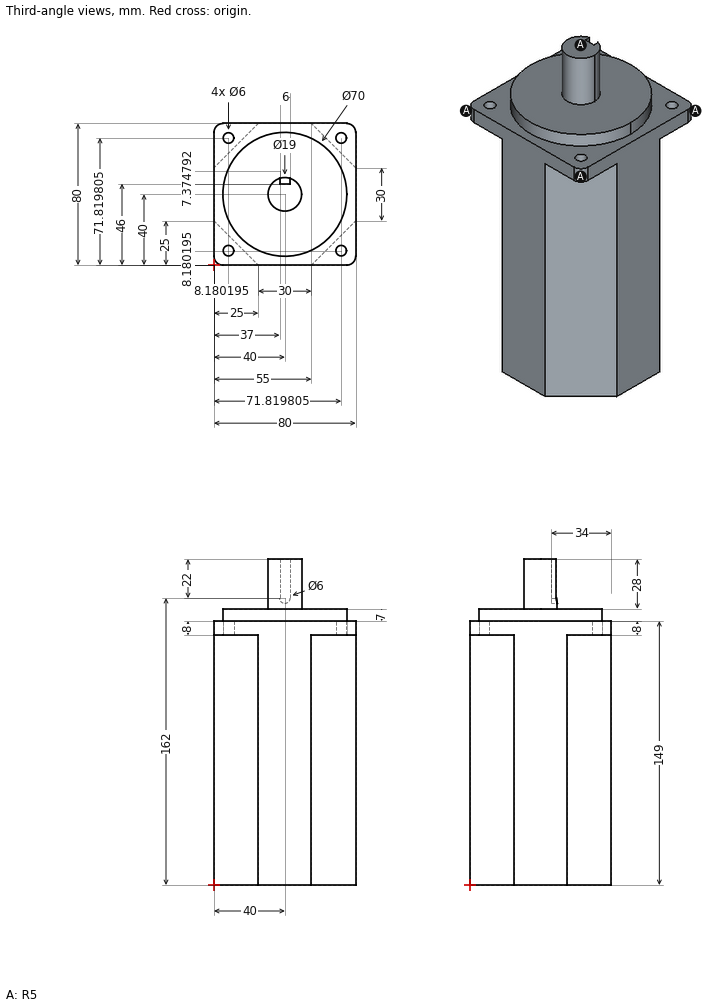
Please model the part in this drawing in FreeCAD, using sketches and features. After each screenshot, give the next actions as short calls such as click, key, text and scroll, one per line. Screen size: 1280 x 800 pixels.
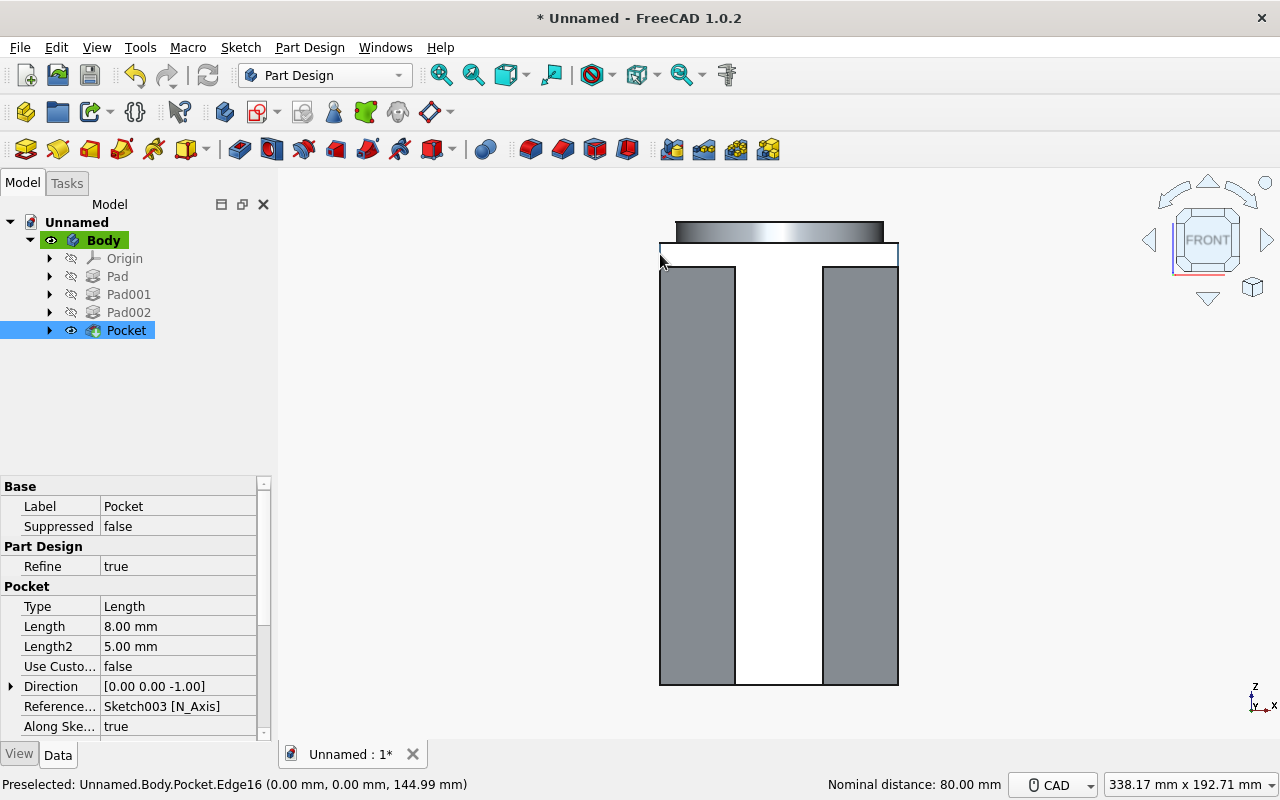
key(3)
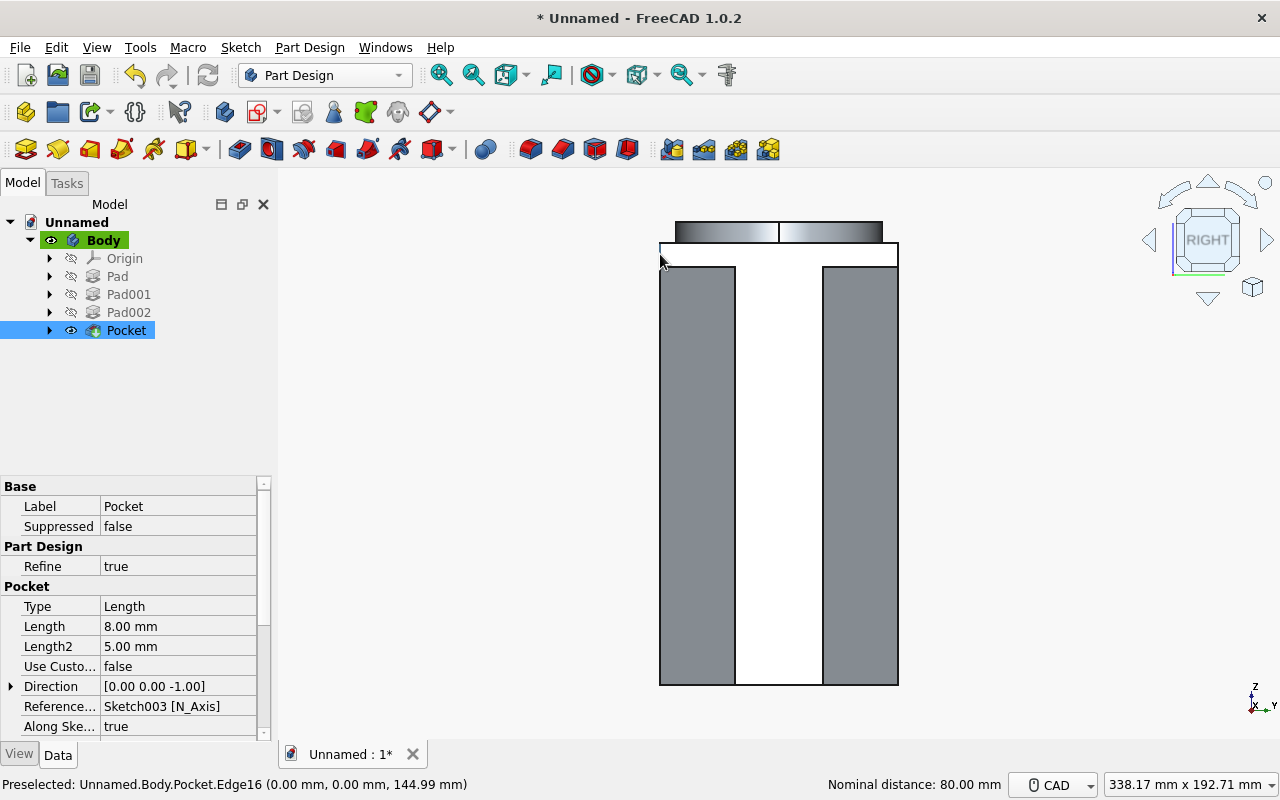
click(898, 254, ctrl)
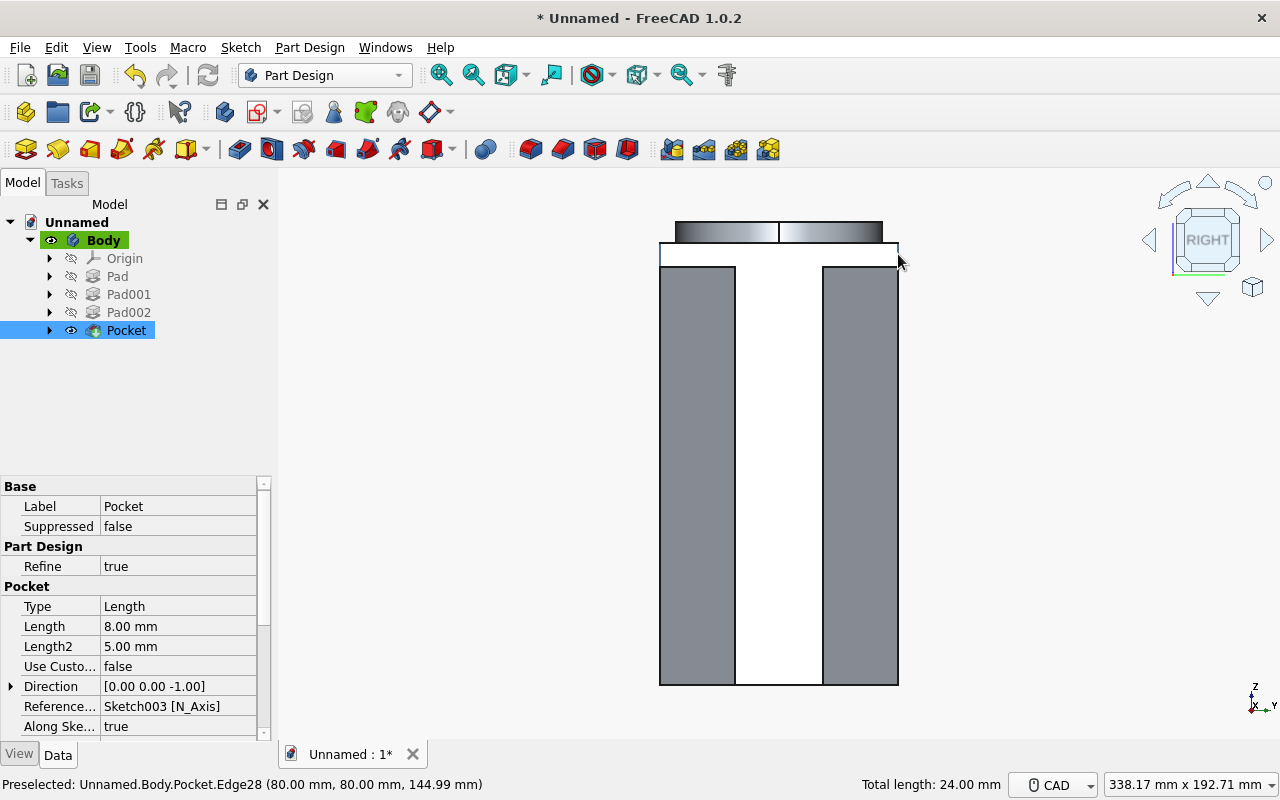
key(5)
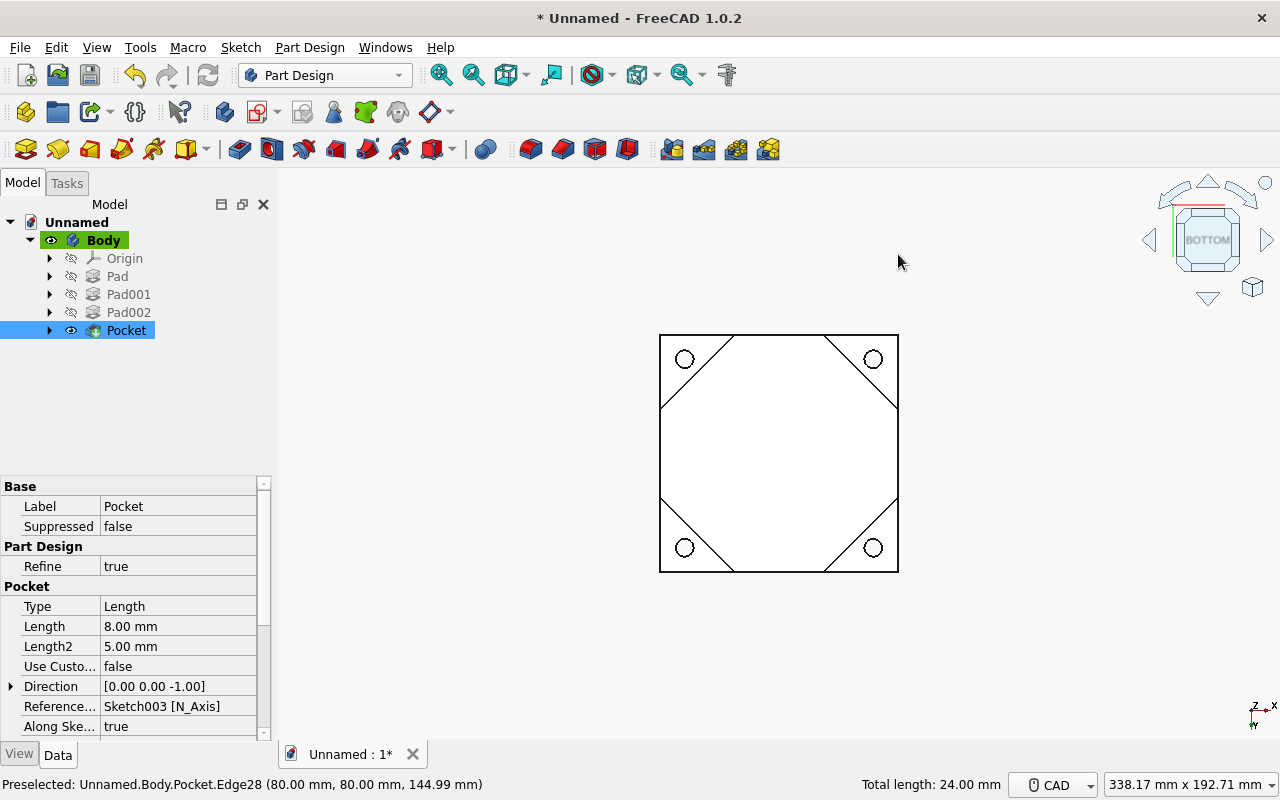
key(v)
key(f)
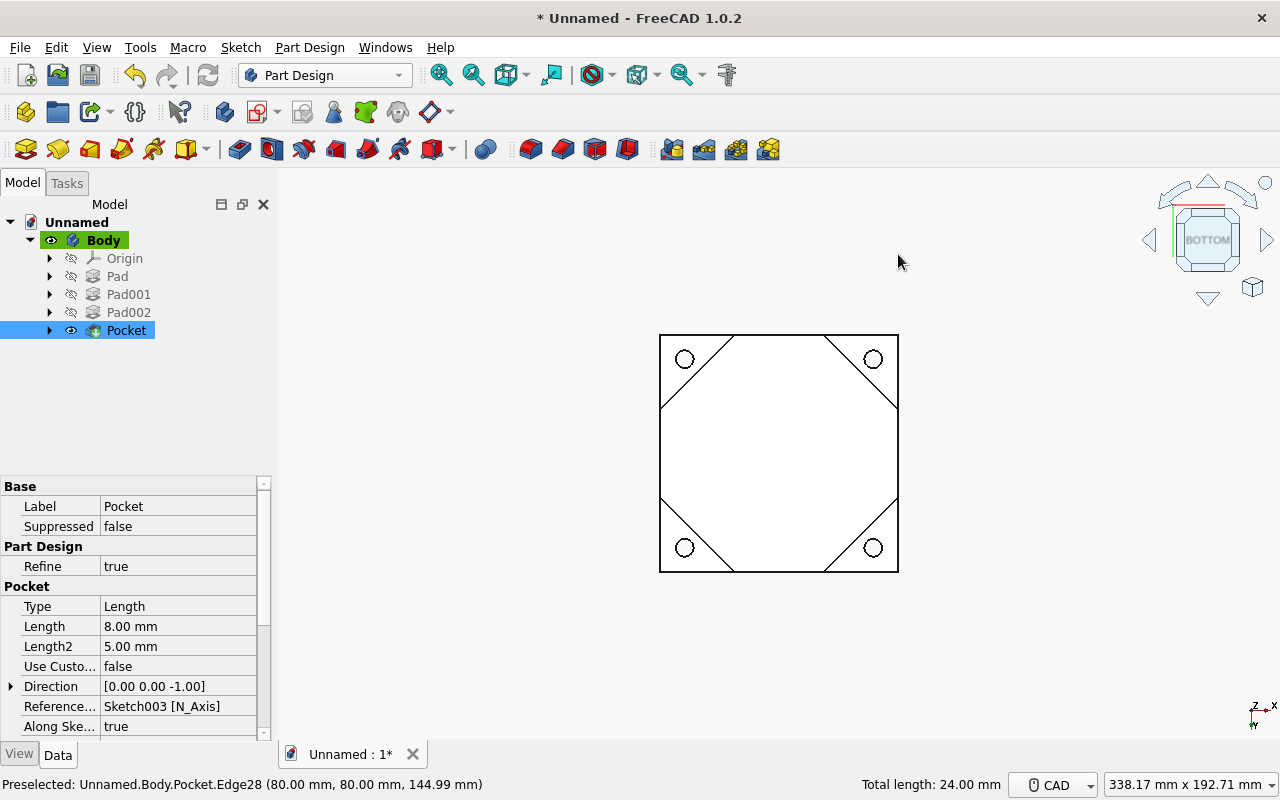
key(4)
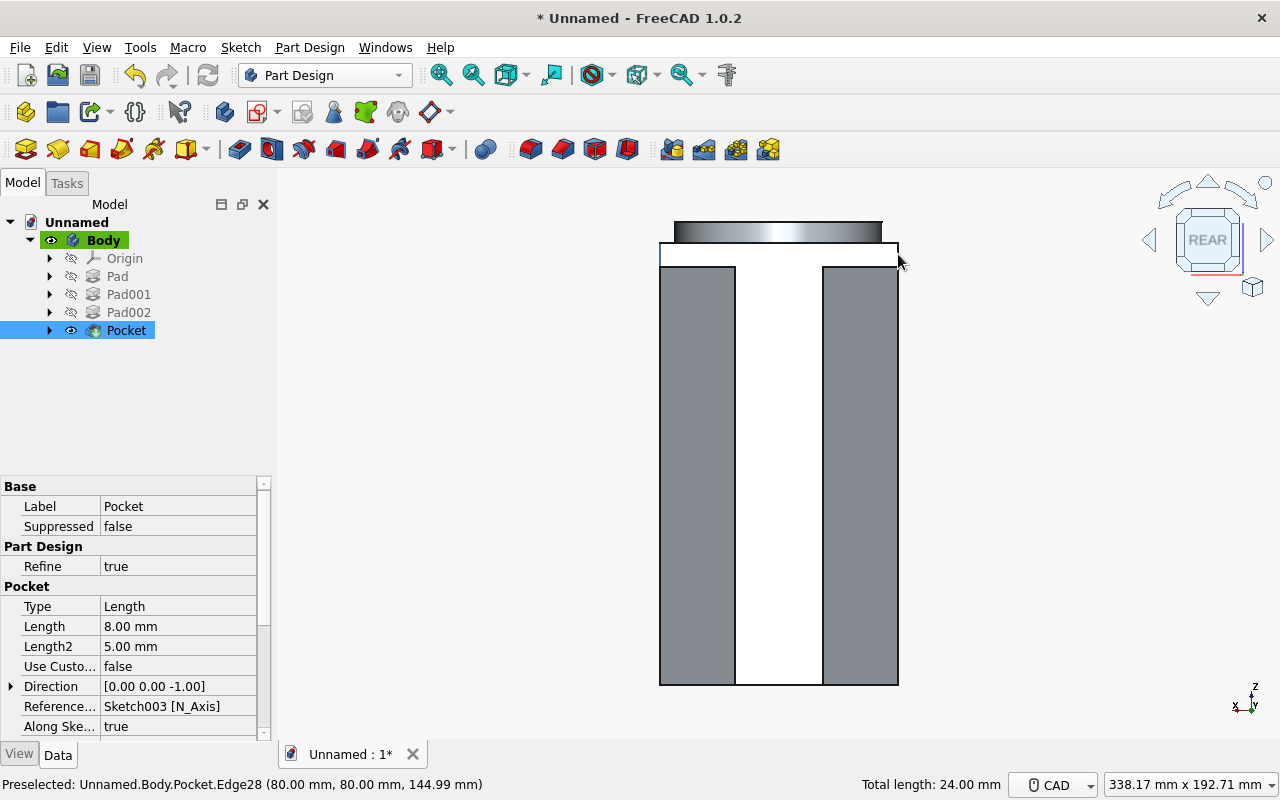
click(898, 254, ctrl)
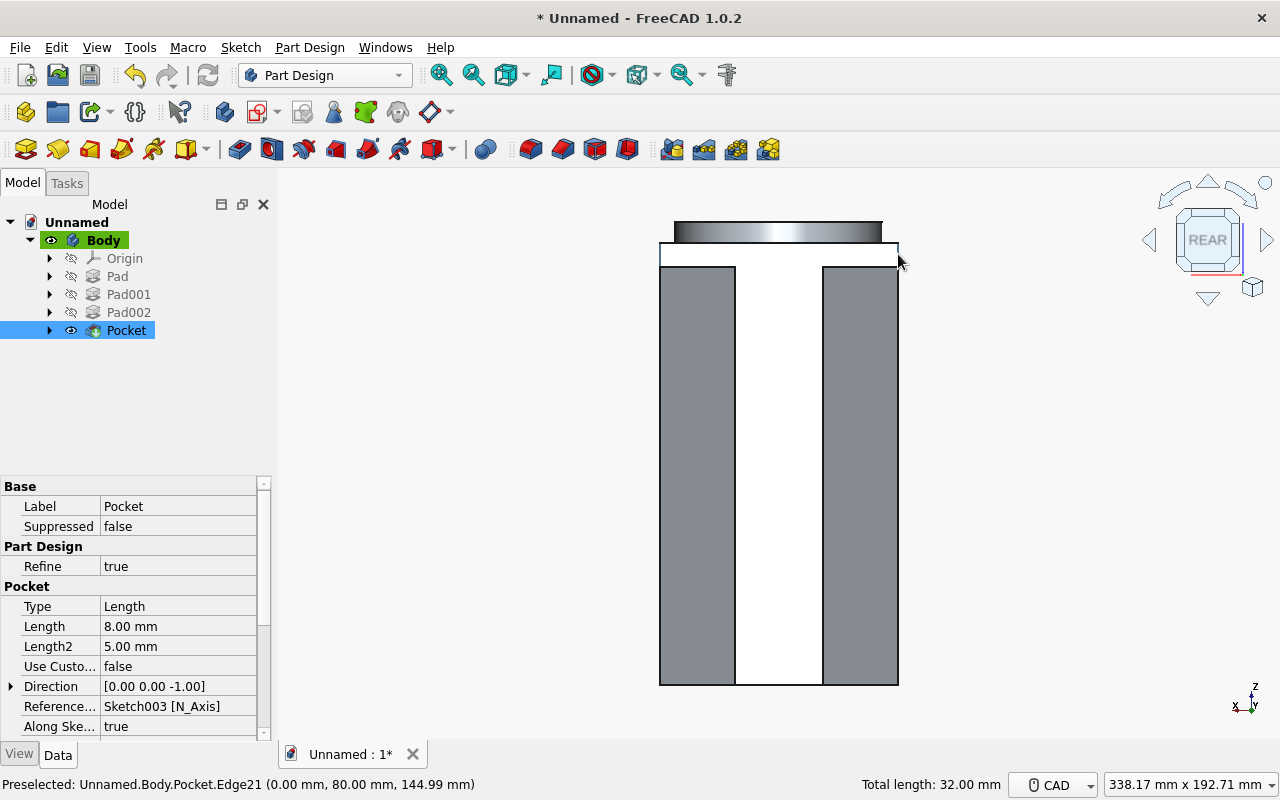
click(532, 150)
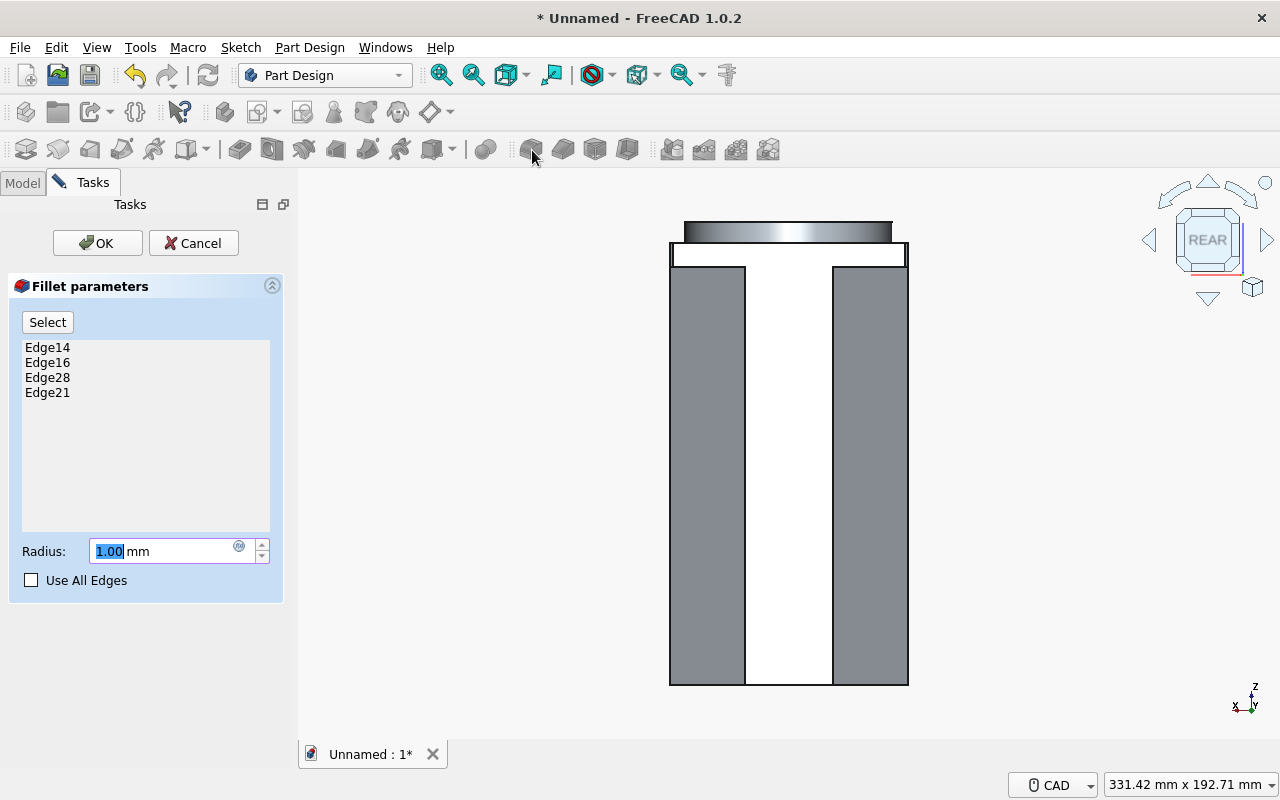
text(5)
key(Tab)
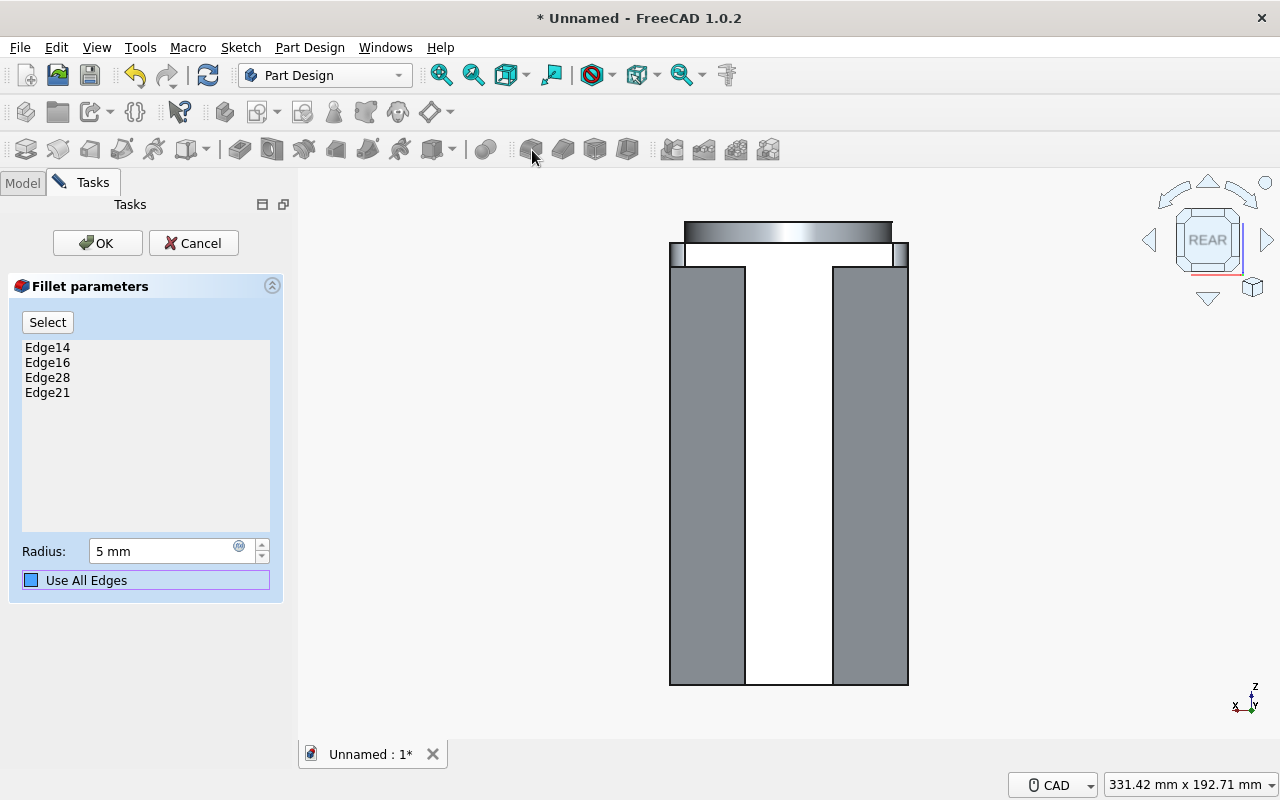
click(98, 243)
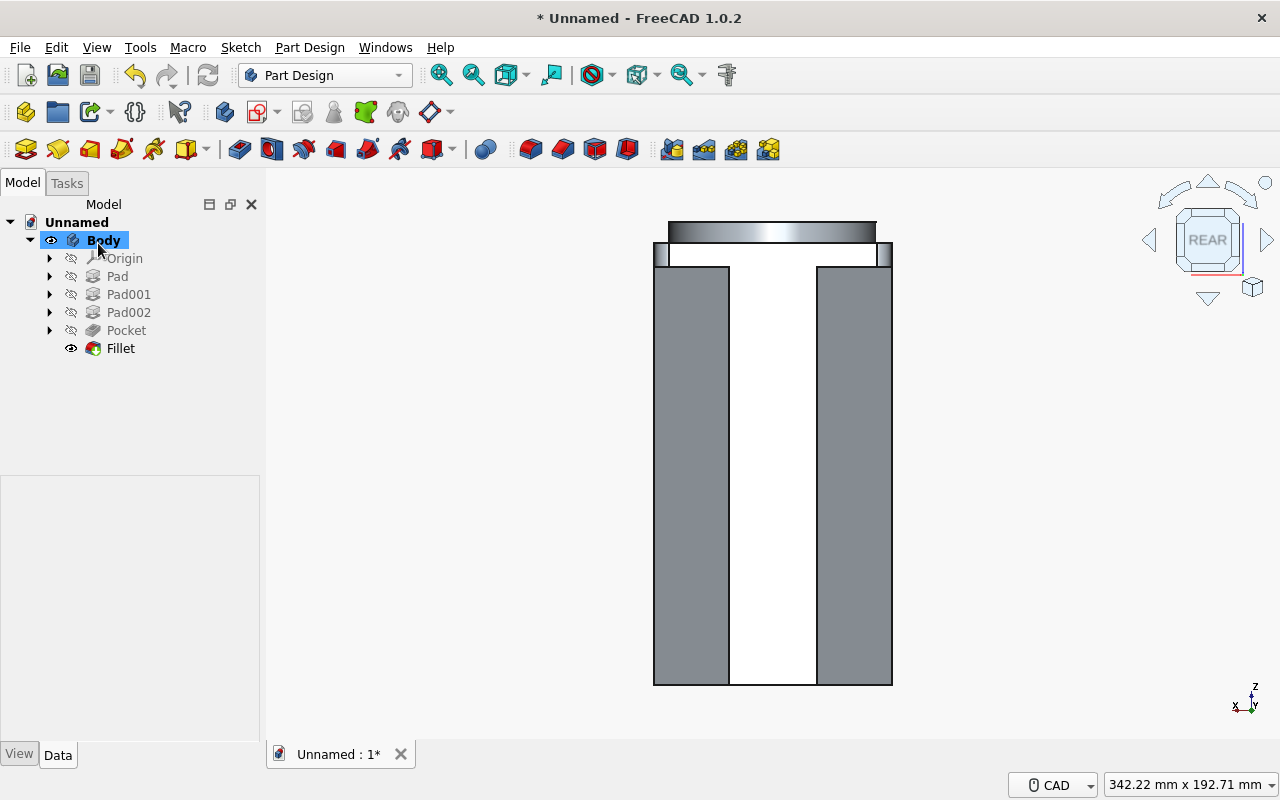
key(0)